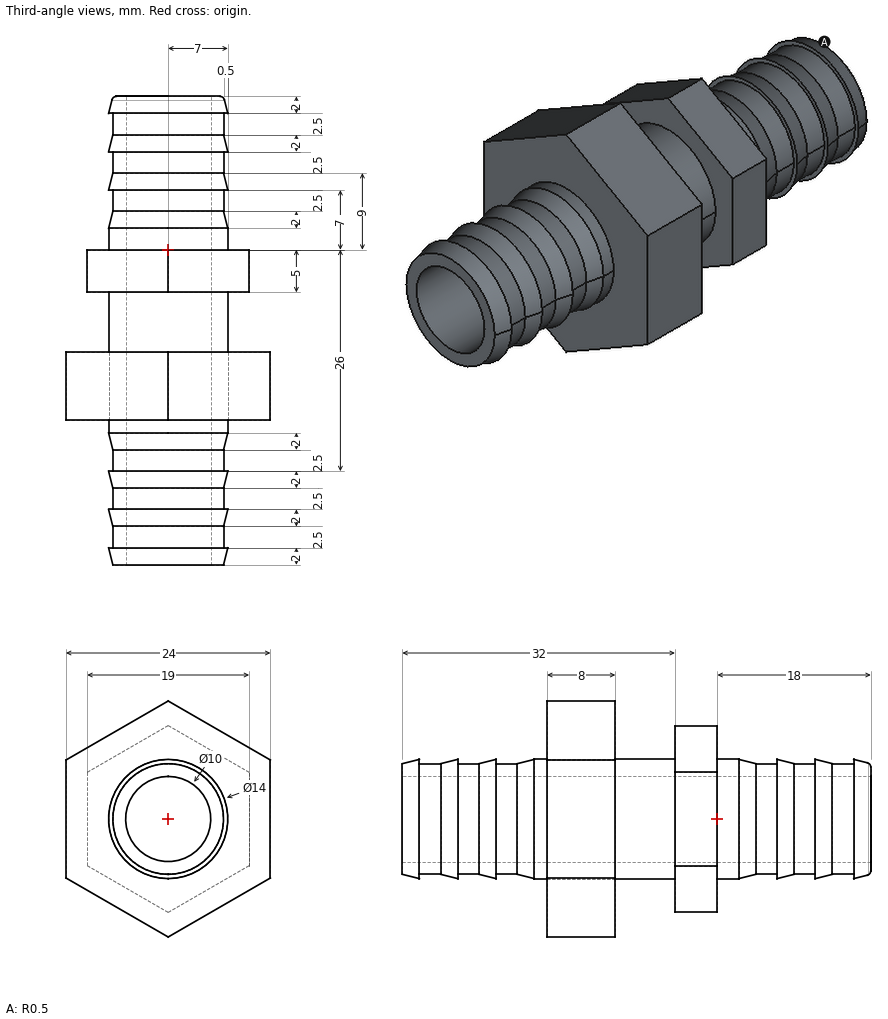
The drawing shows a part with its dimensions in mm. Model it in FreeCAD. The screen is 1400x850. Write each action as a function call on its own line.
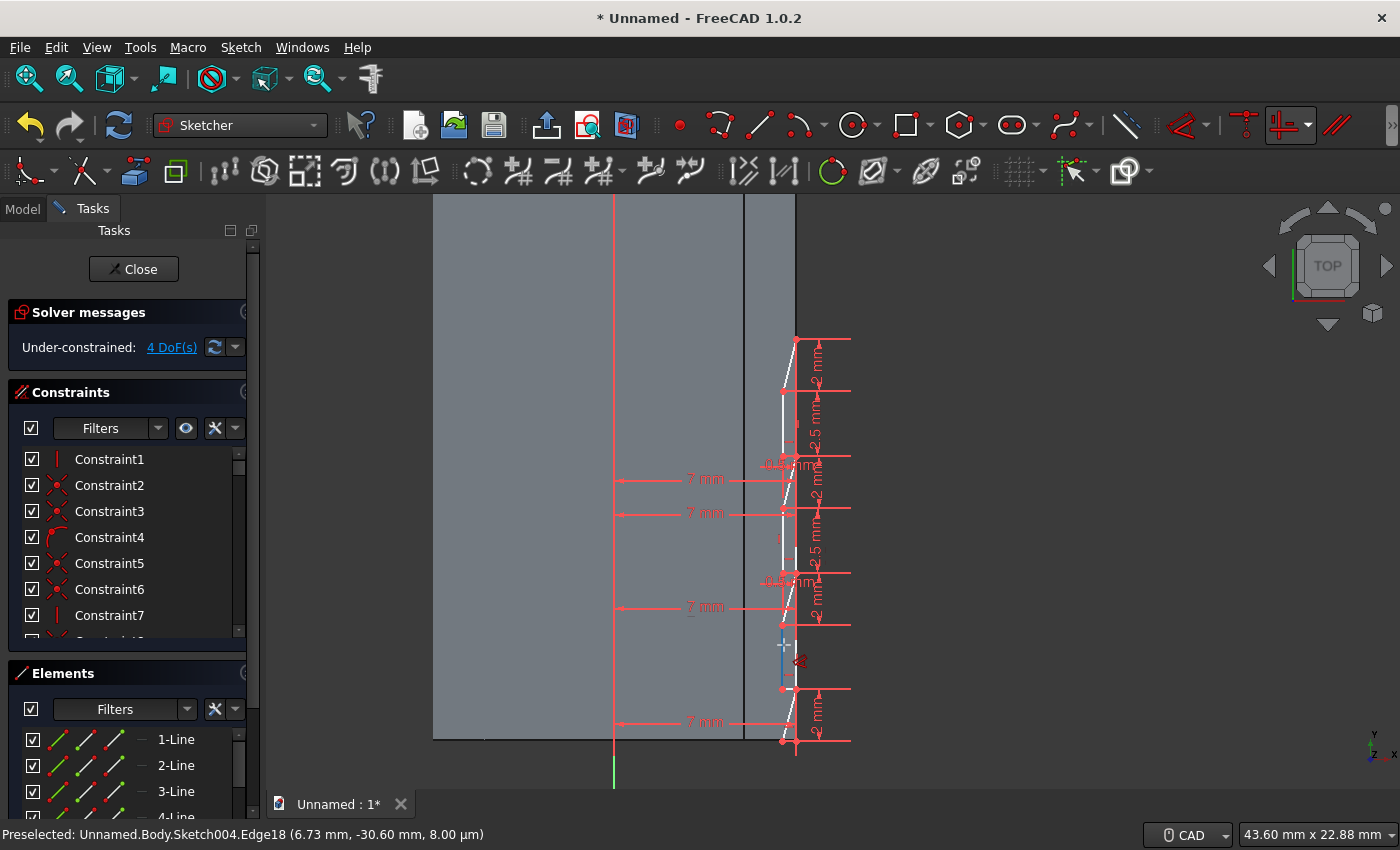
click(782, 645)
click(816, 657)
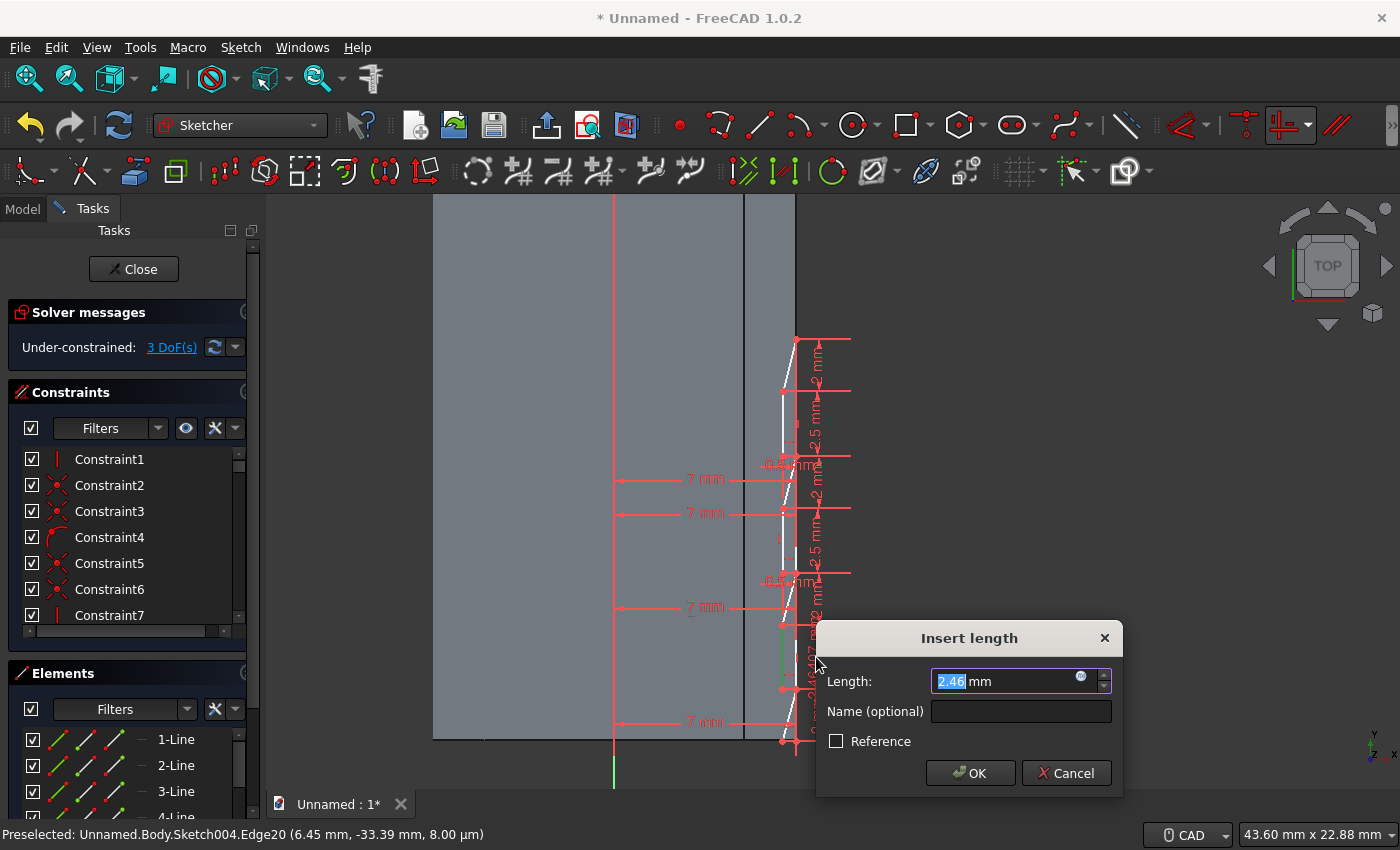
text(2.5)
key(Return)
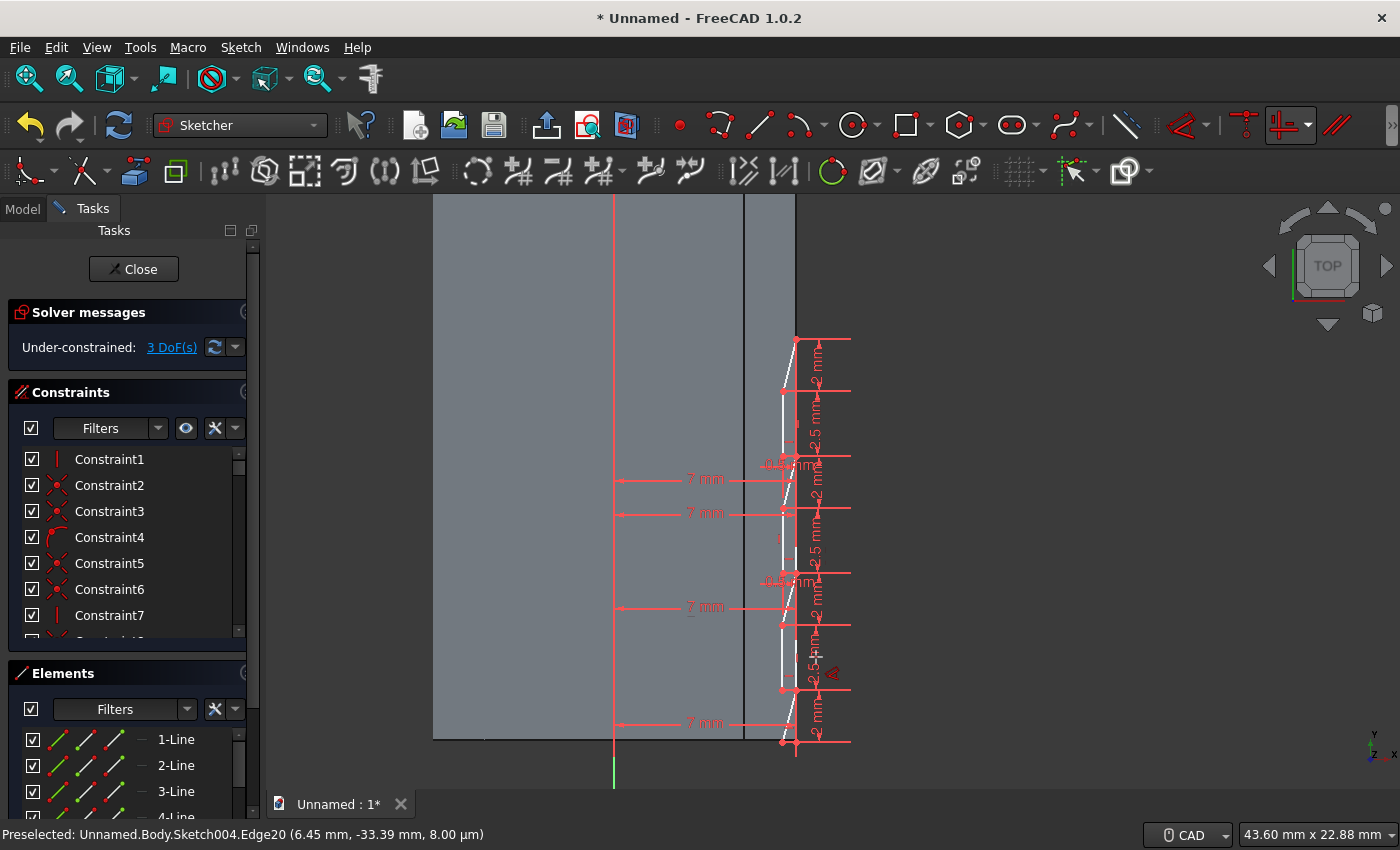
scroll(789, 690, up, 6)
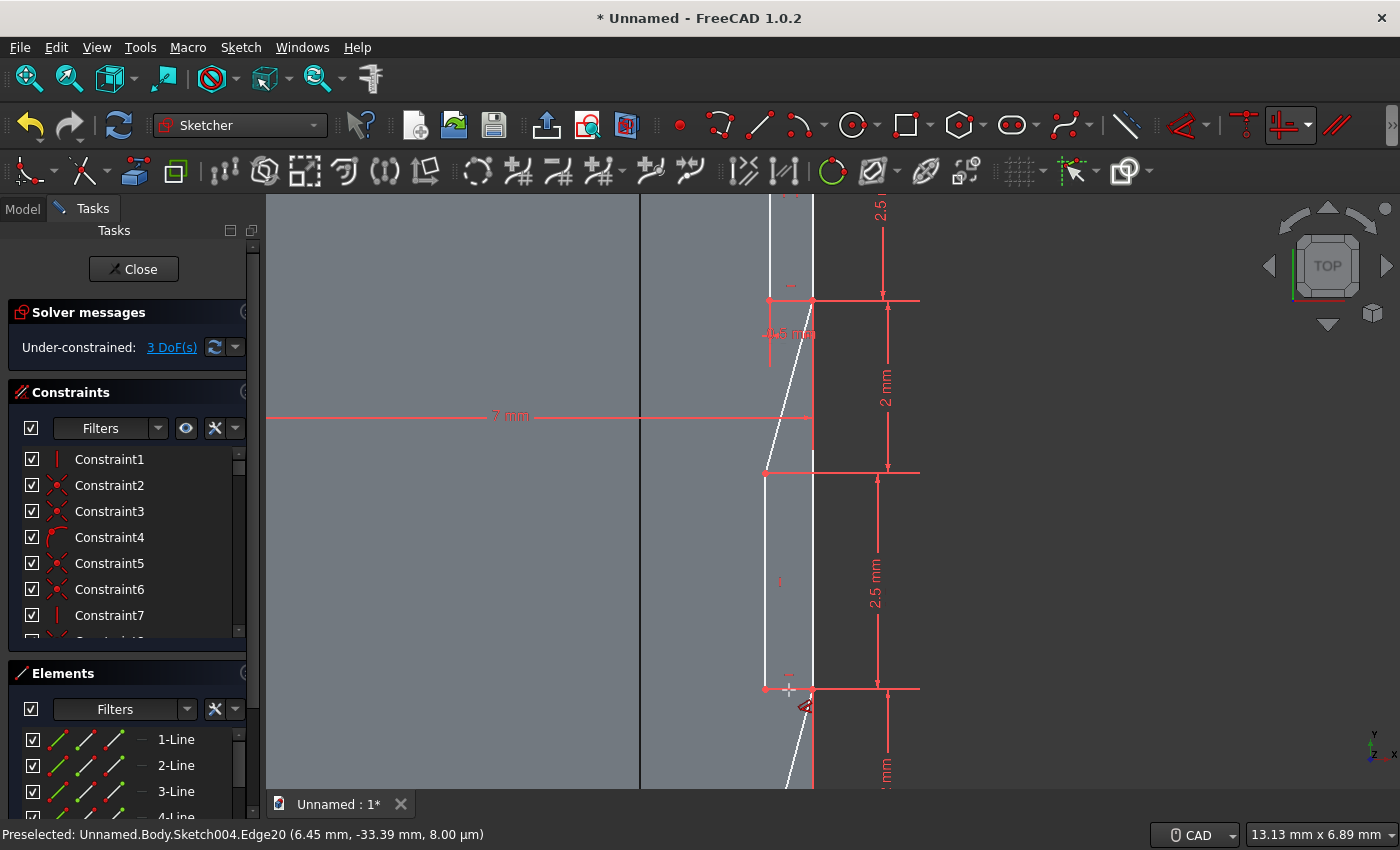
click(789, 689)
click(789, 723)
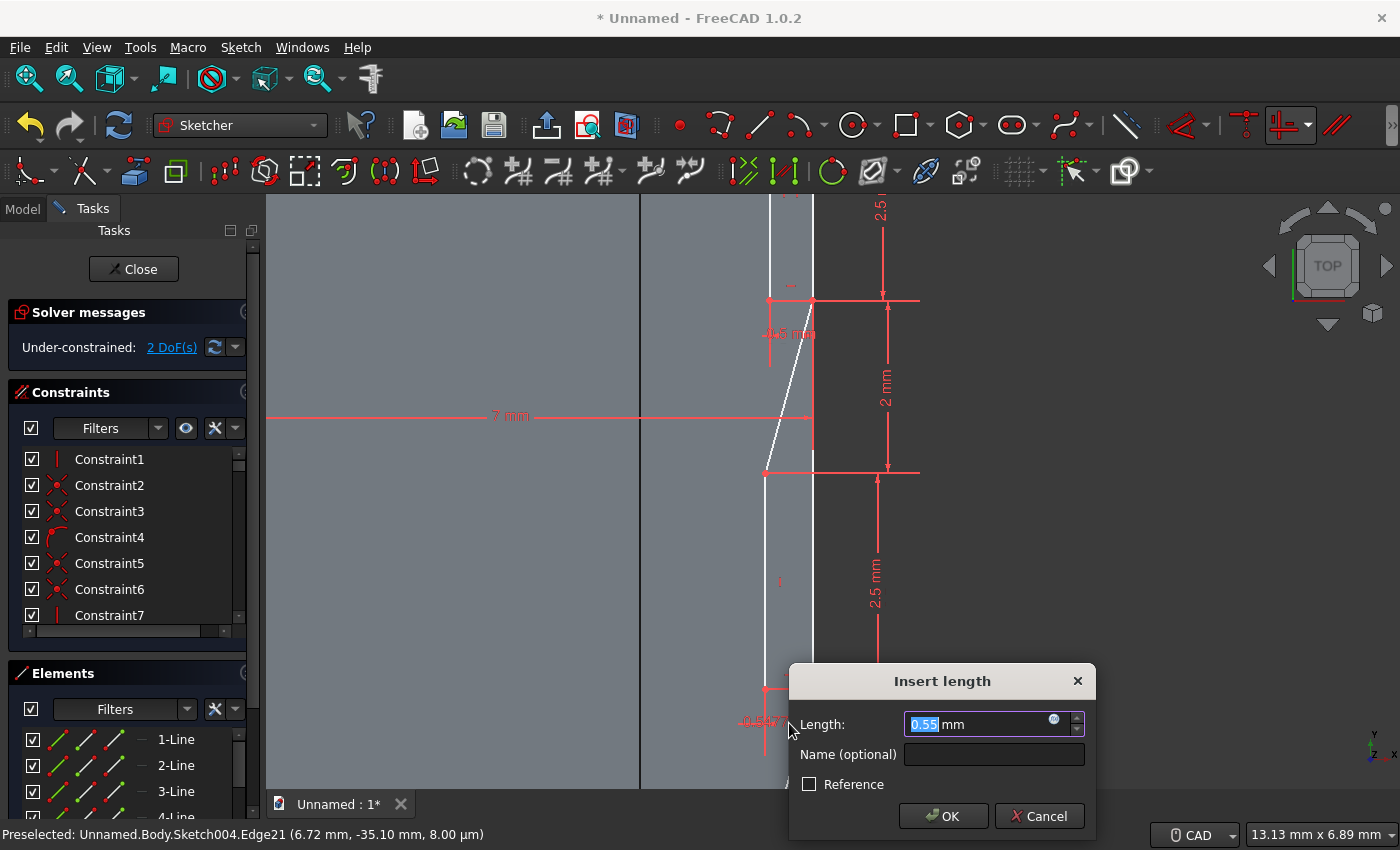
text(0.5)
key(Return)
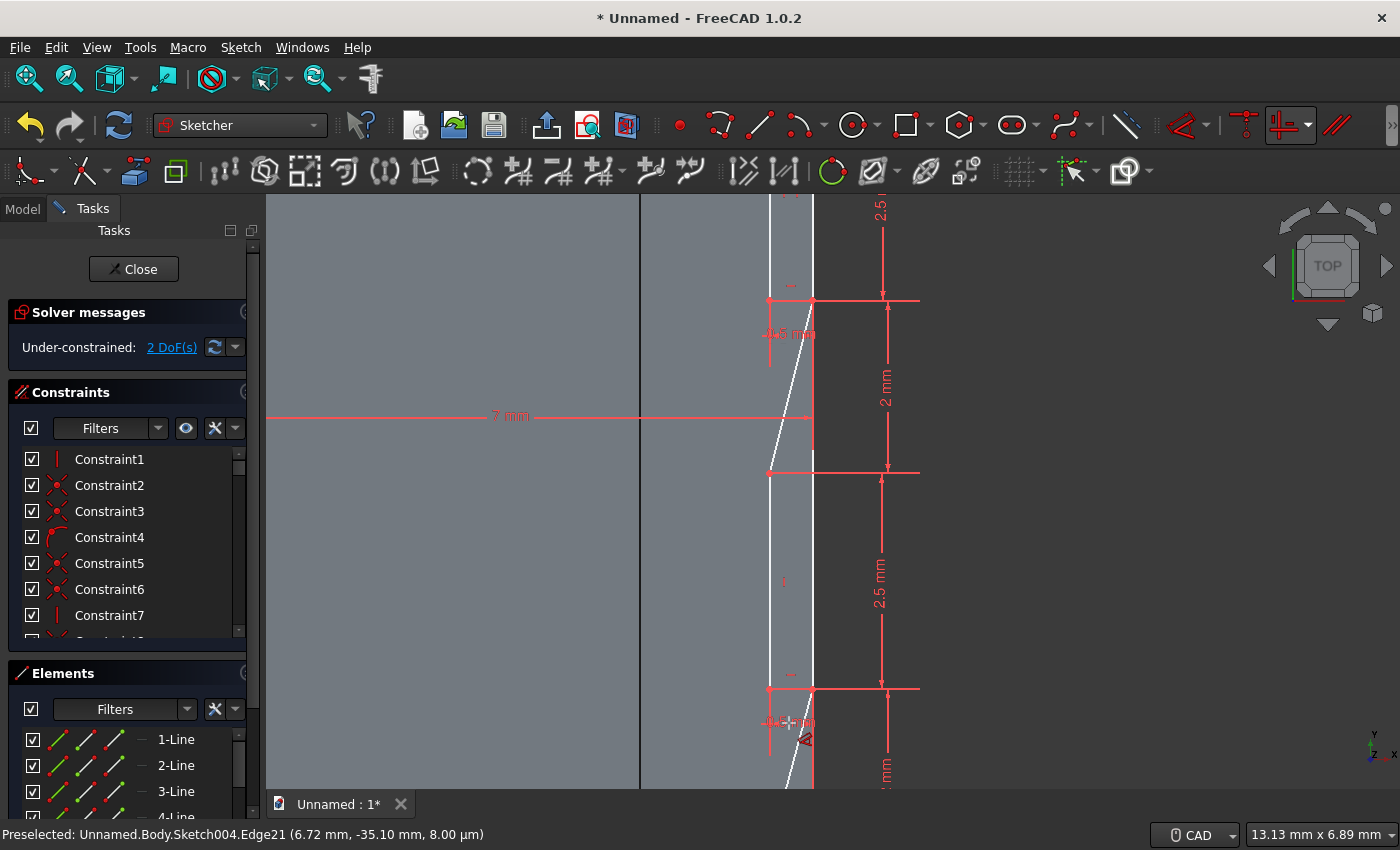
scroll(785, 653, down, 13)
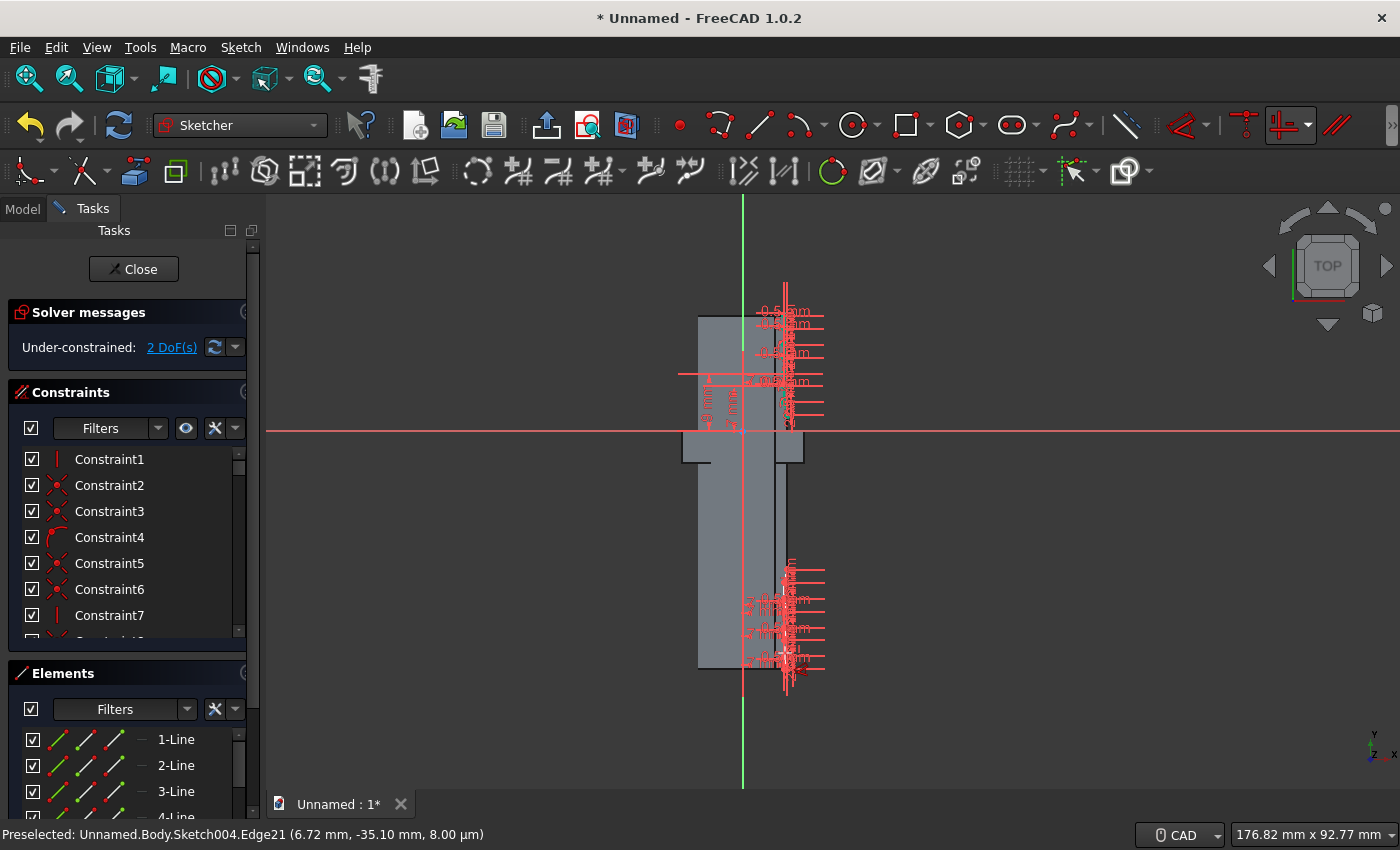
scroll(785, 669, up, 14)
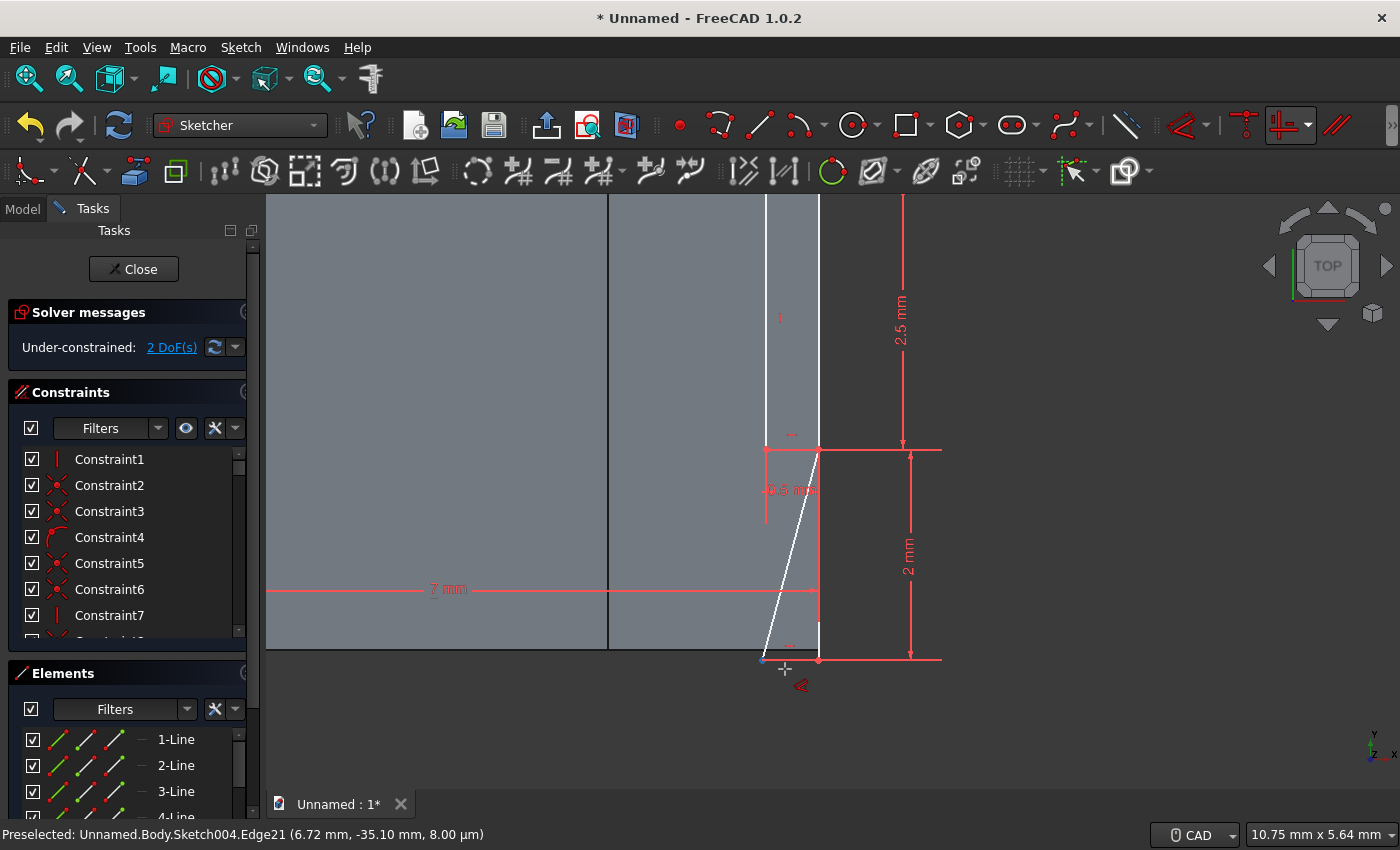
click(779, 660)
click(791, 694)